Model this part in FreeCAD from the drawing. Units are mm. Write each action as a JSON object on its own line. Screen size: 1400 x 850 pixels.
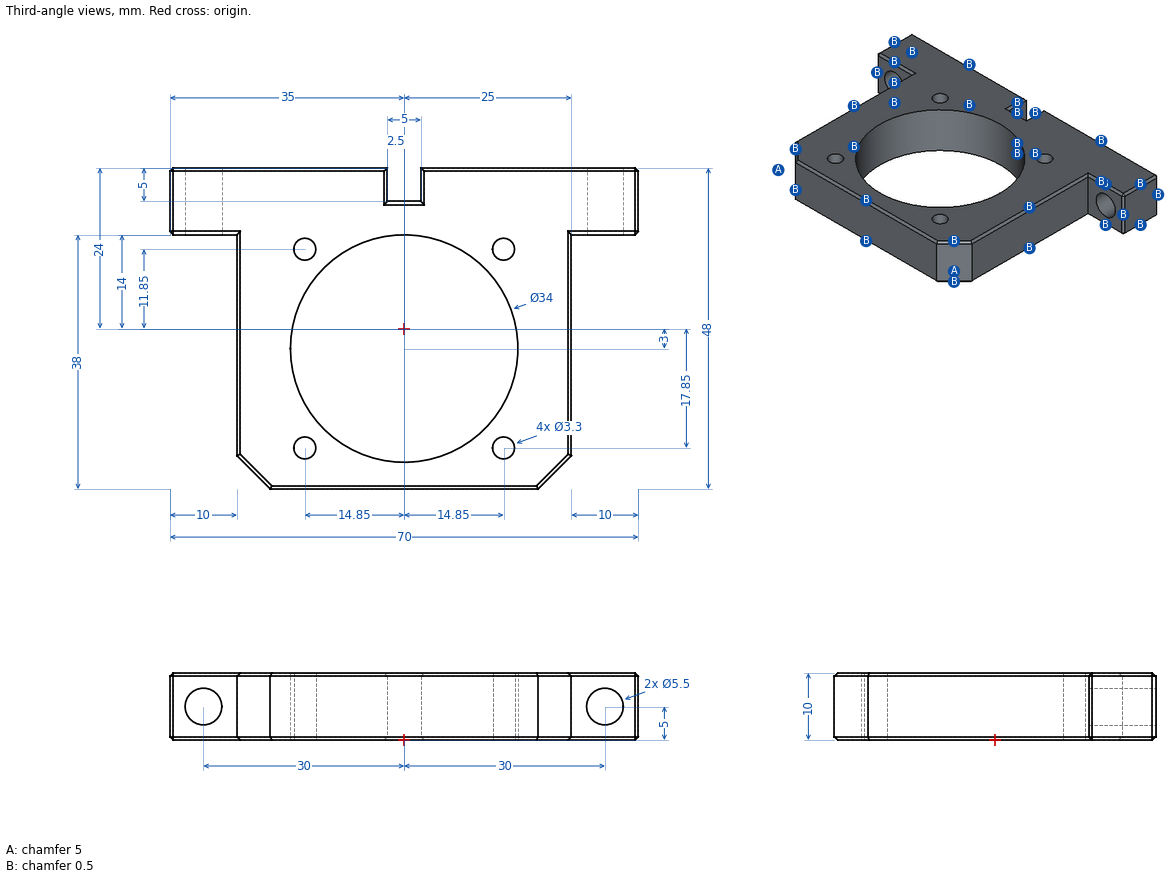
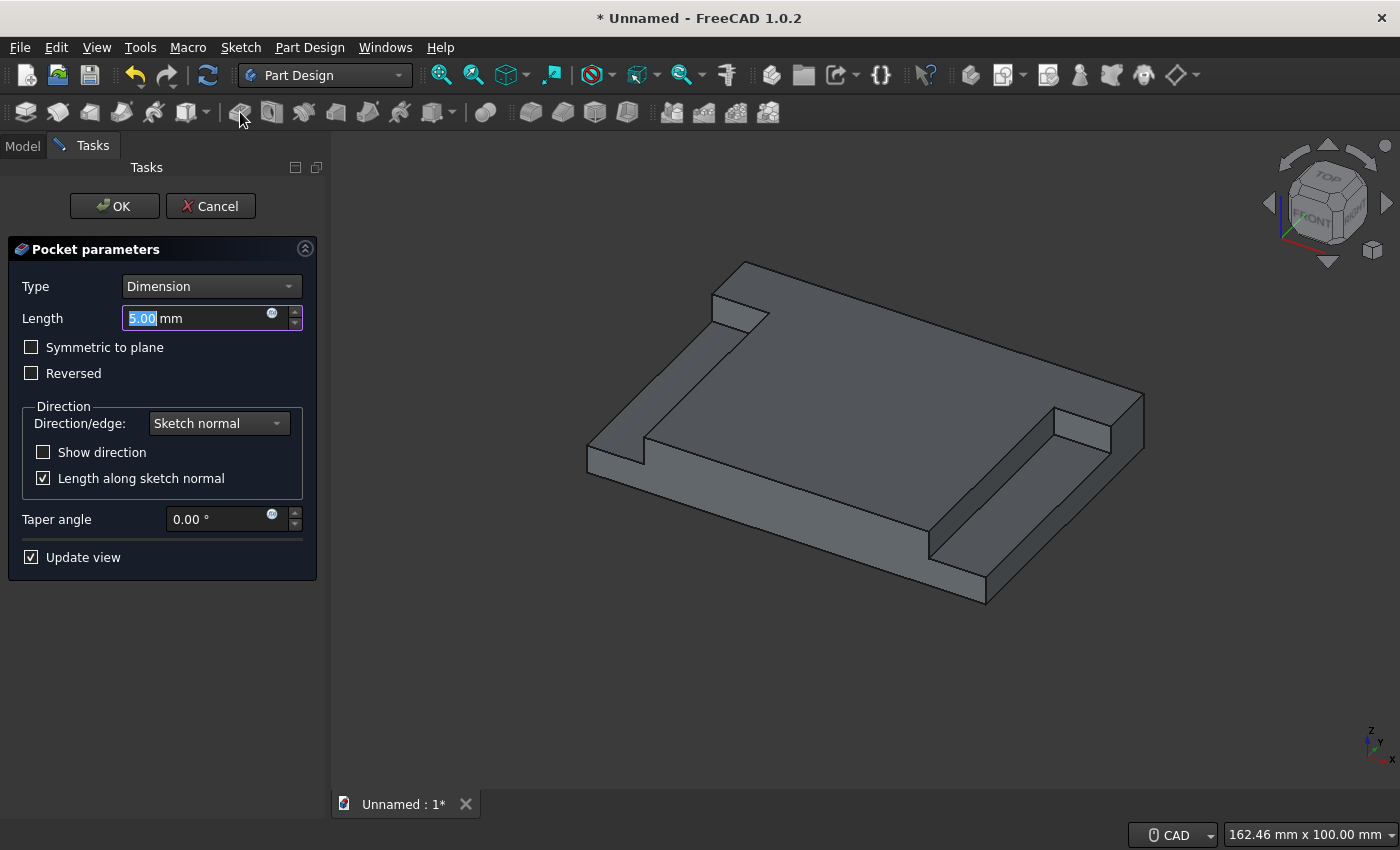
{"action": "left_click", "coordinate": [212, 286]}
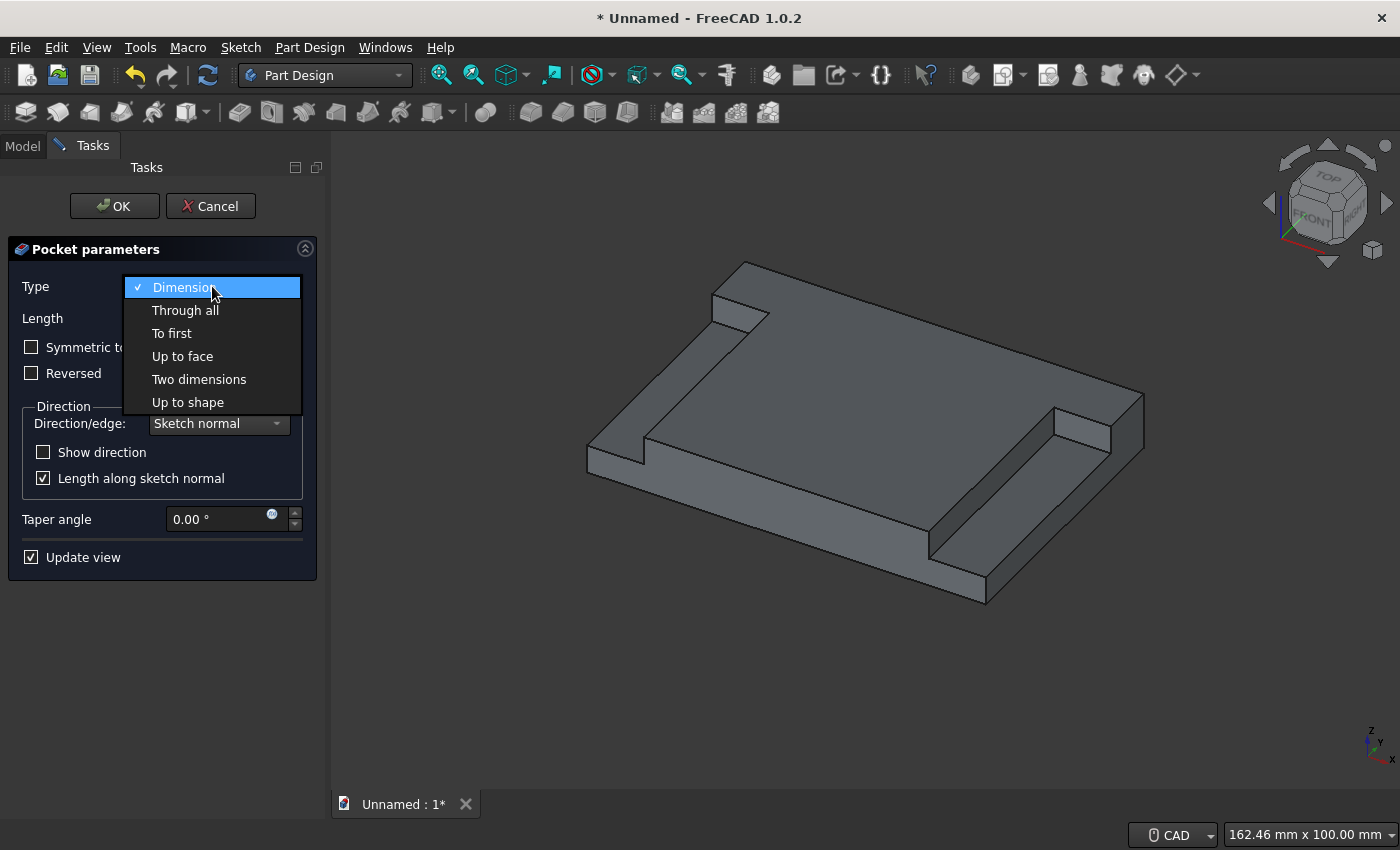
{"action": "left_click", "coordinate": [212, 310]}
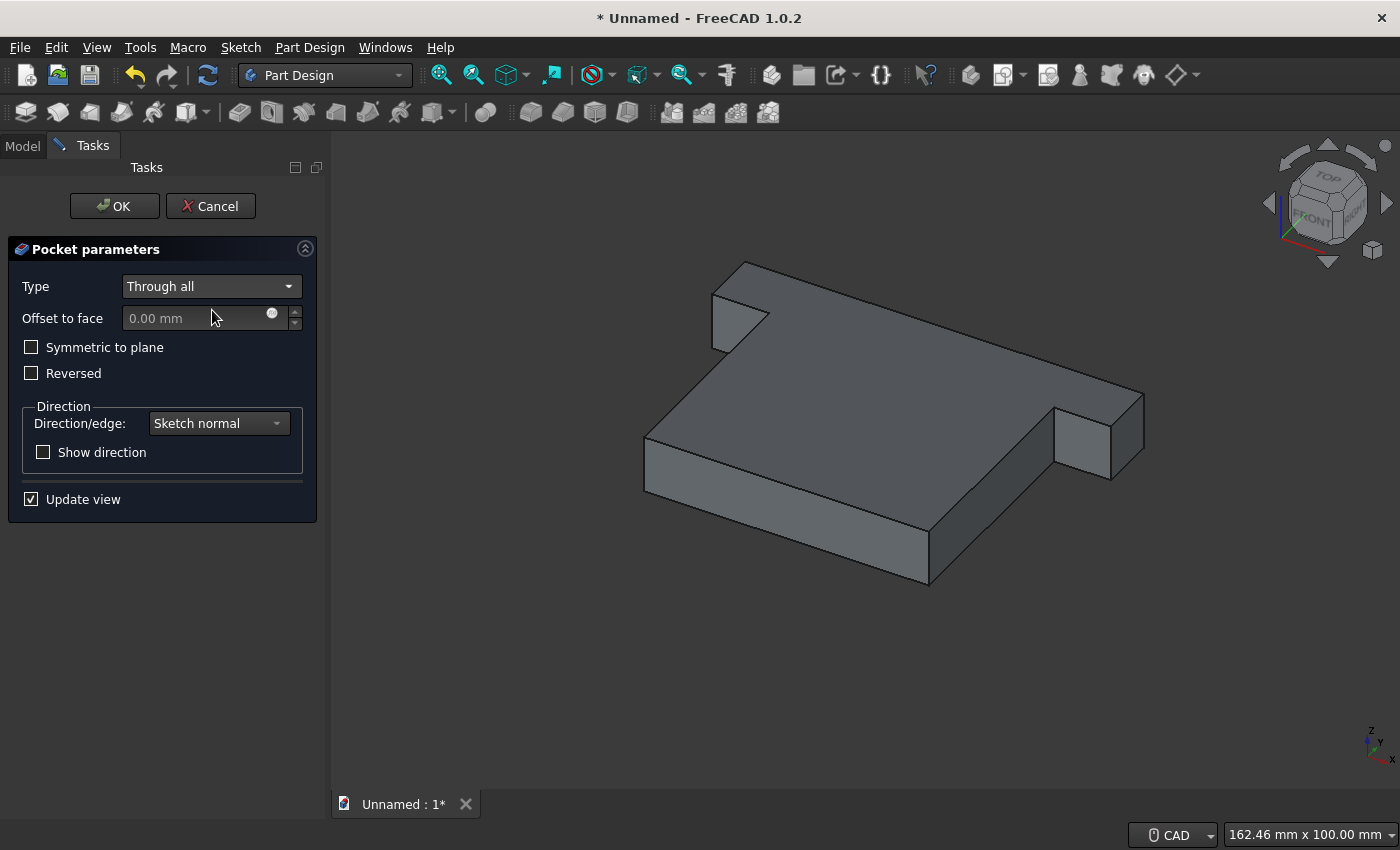
{"action": "left_click", "coordinate": [115, 206]}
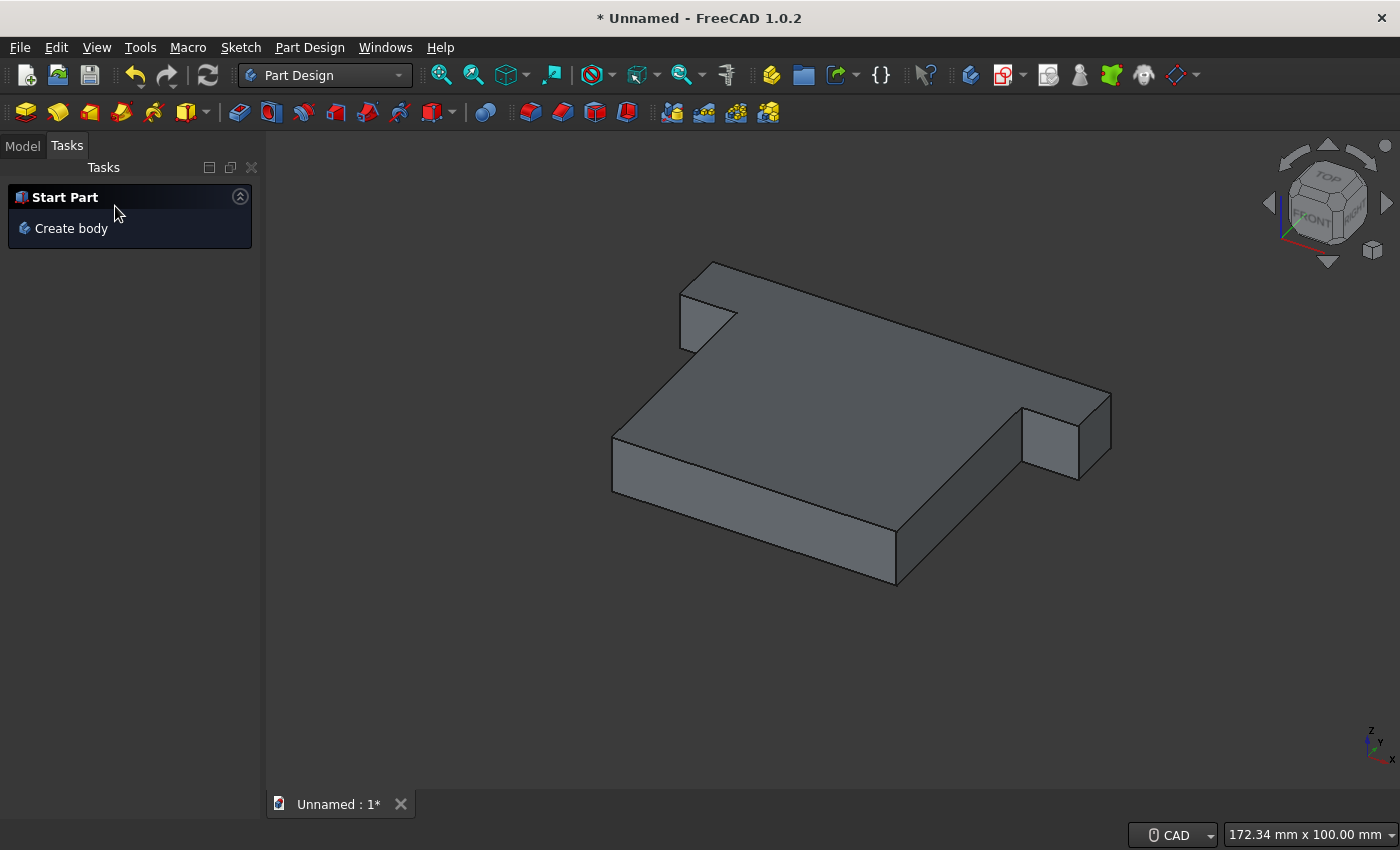
{"action": "left_click", "coordinate": [1004, 76]}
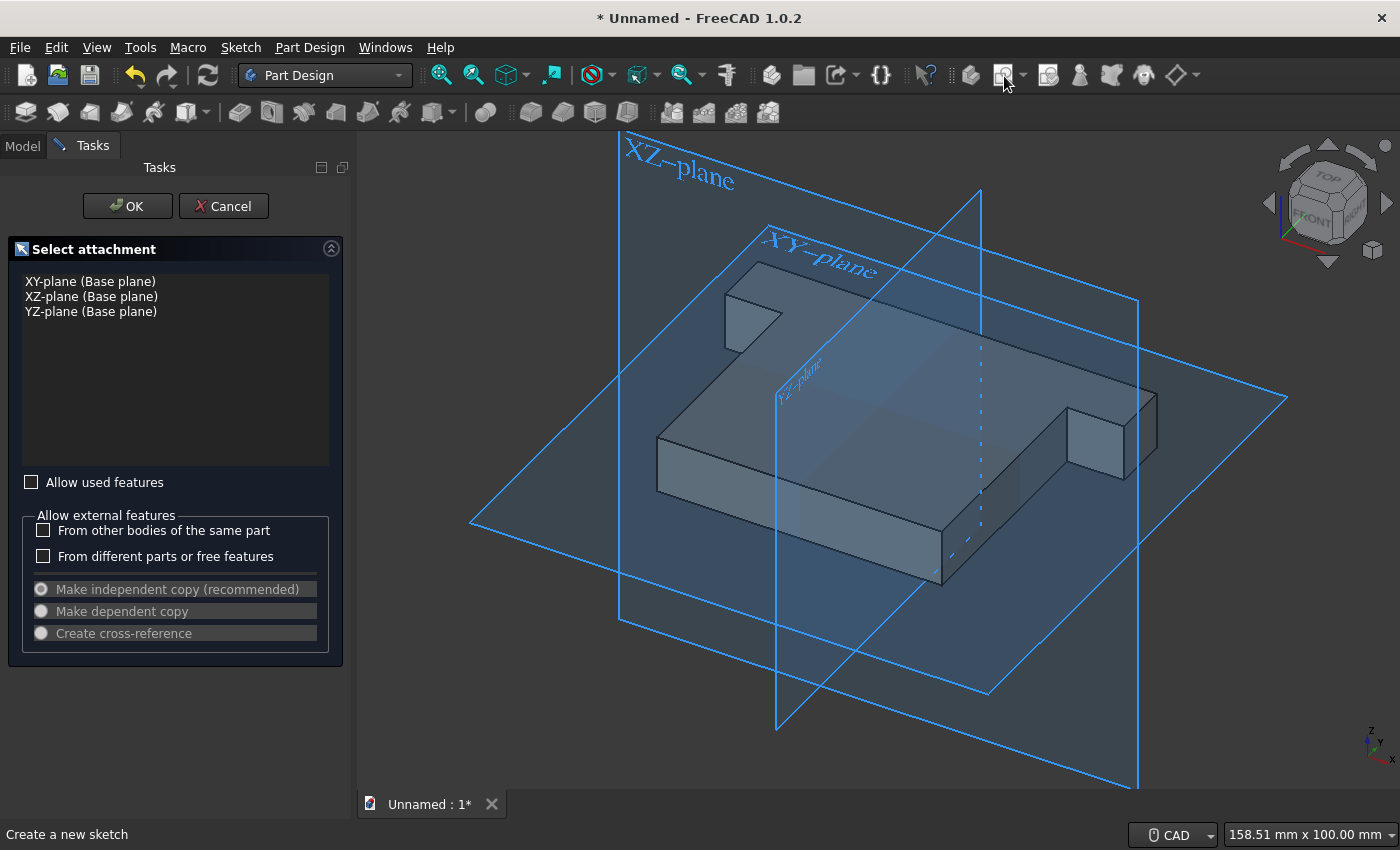
{"action": "left_click", "coordinate": [82, 282]}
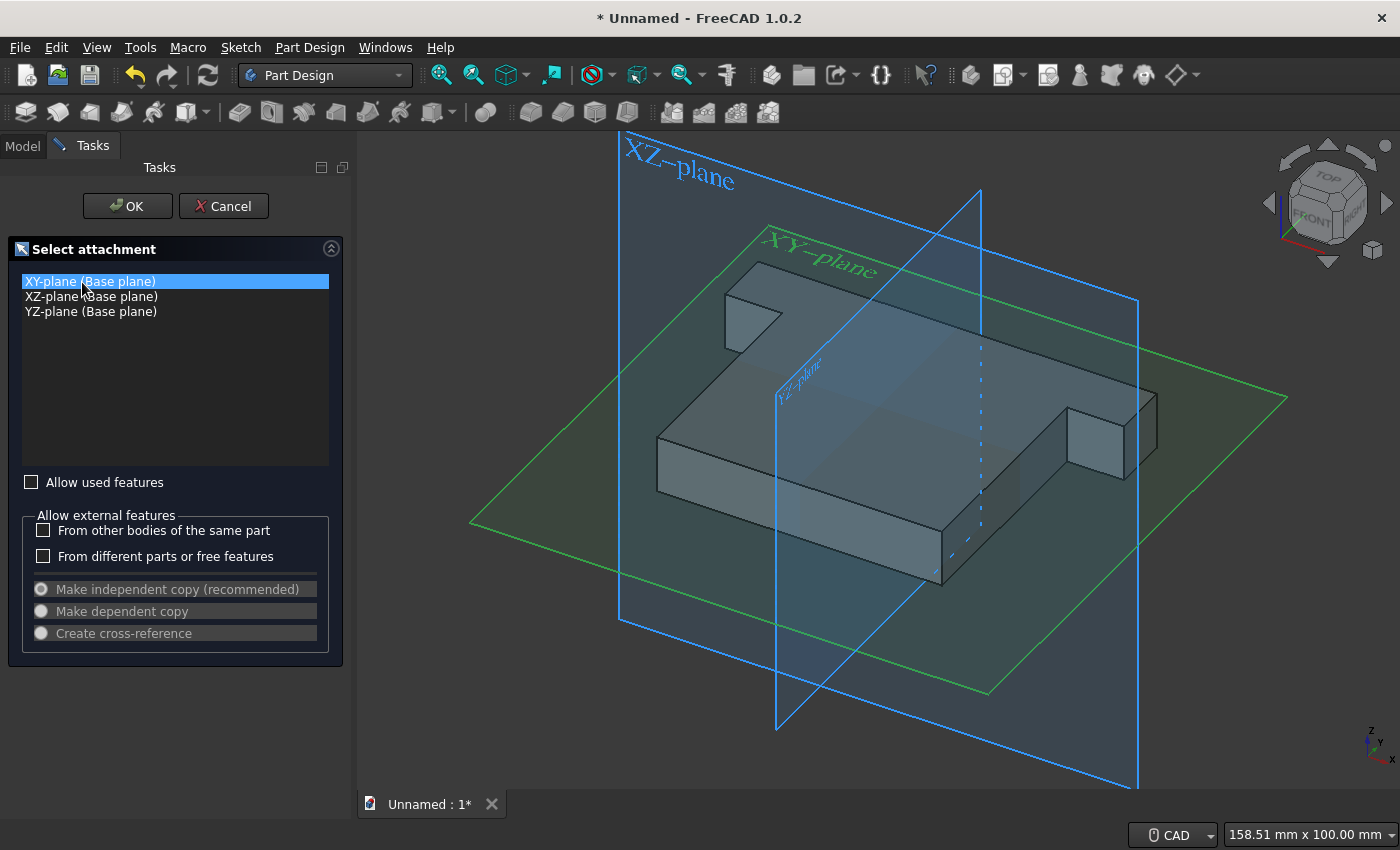
{"action": "left_click", "coordinate": [128, 206]}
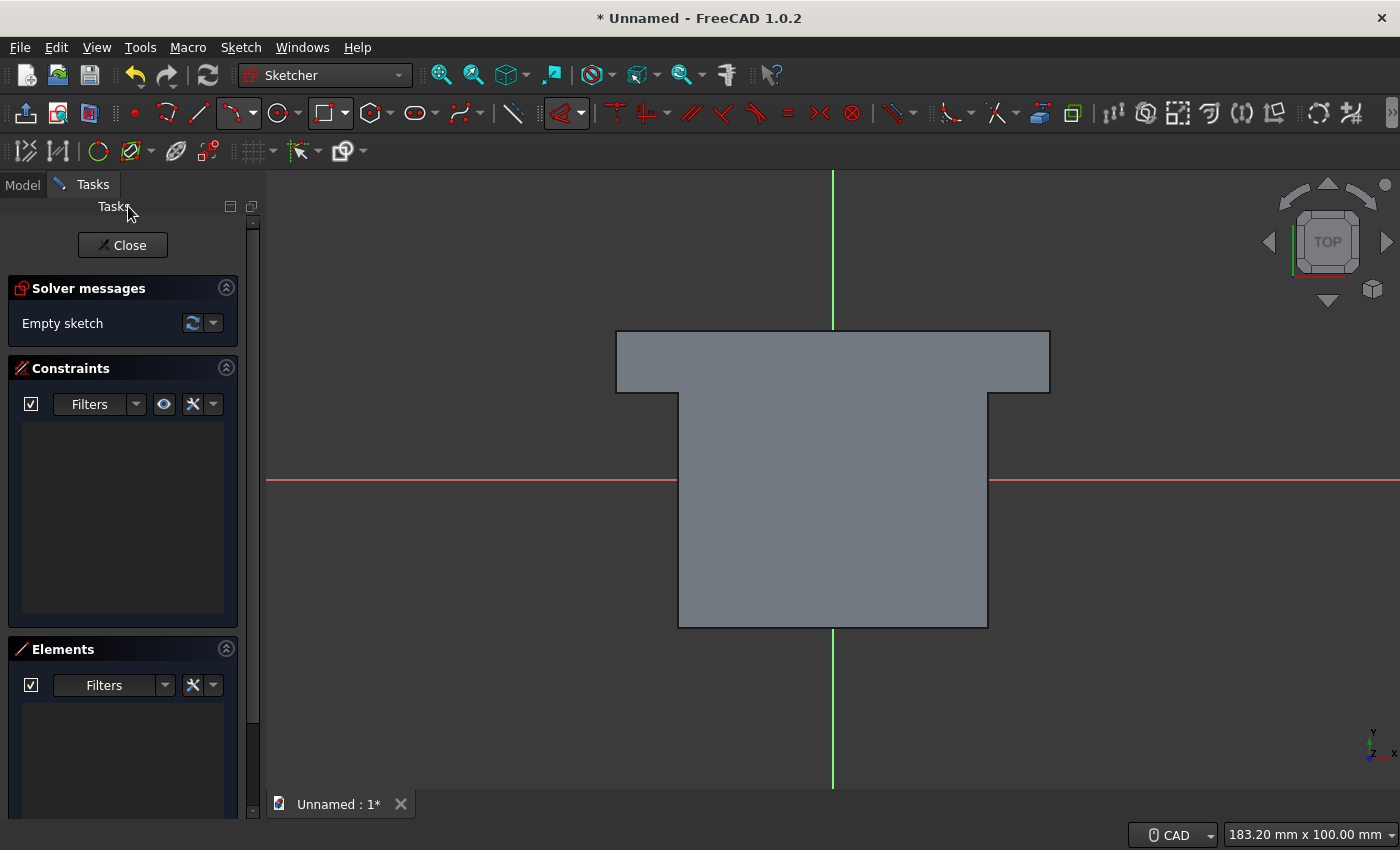
{"action": "left_click", "coordinate": [90, 114]}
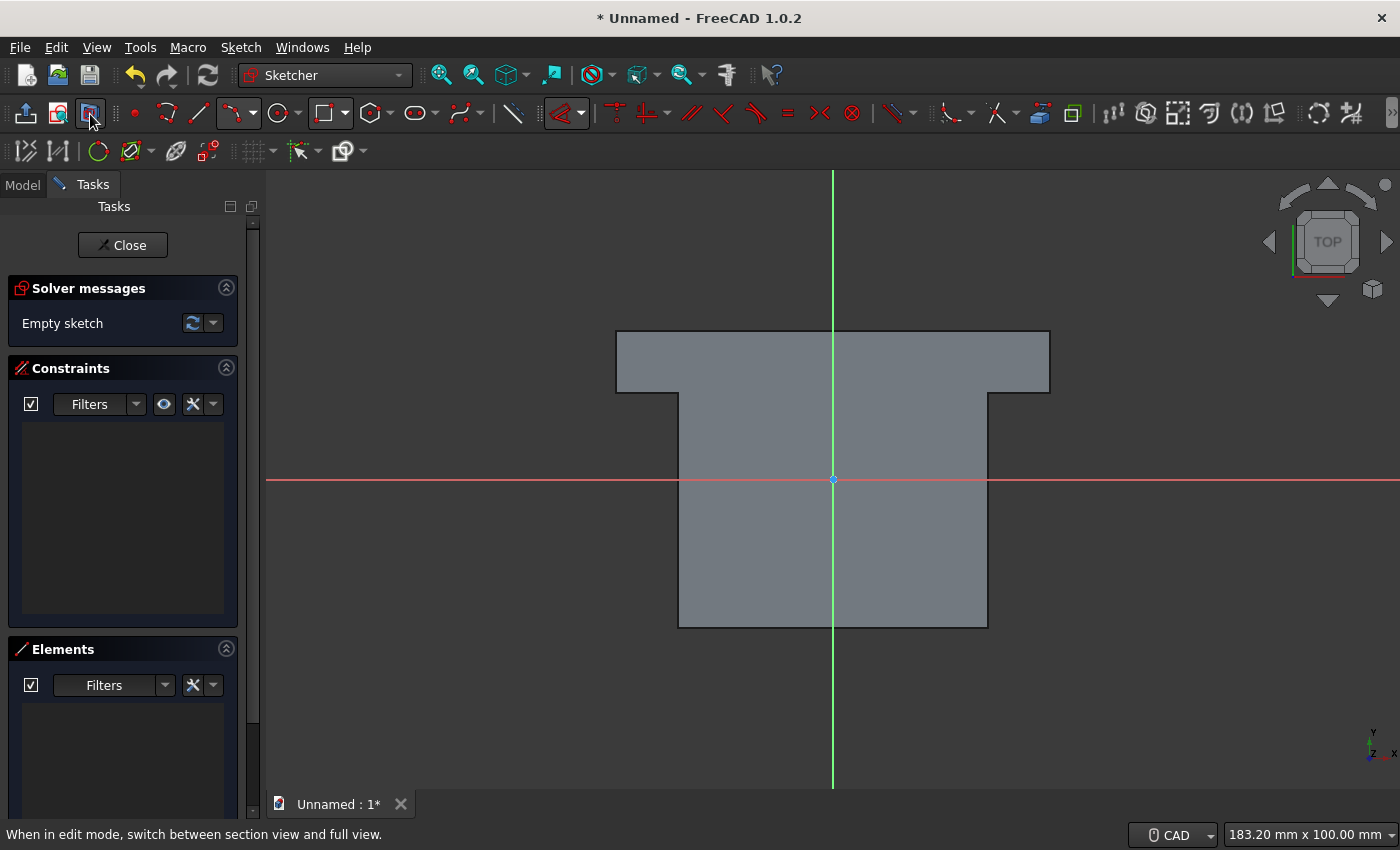
{"action": "scroll", "coordinate": [916, 521], "scroll_direction": "up", "scroll_amount": 3}